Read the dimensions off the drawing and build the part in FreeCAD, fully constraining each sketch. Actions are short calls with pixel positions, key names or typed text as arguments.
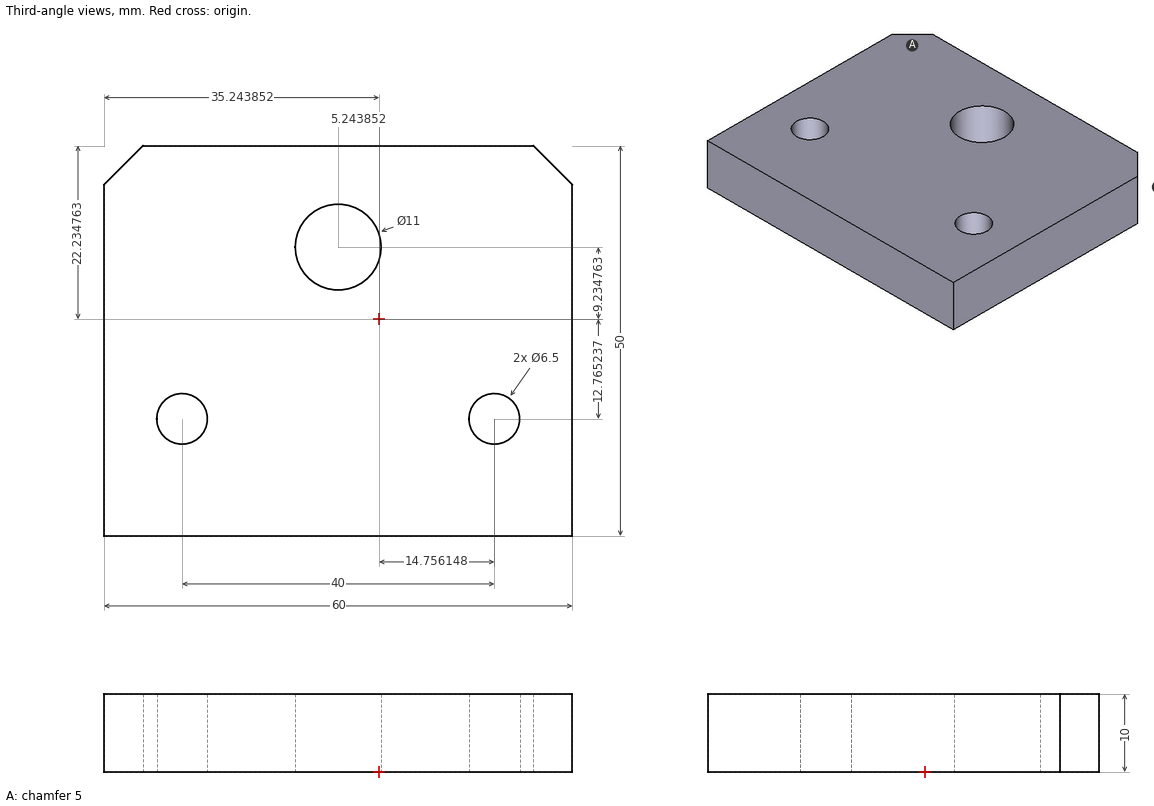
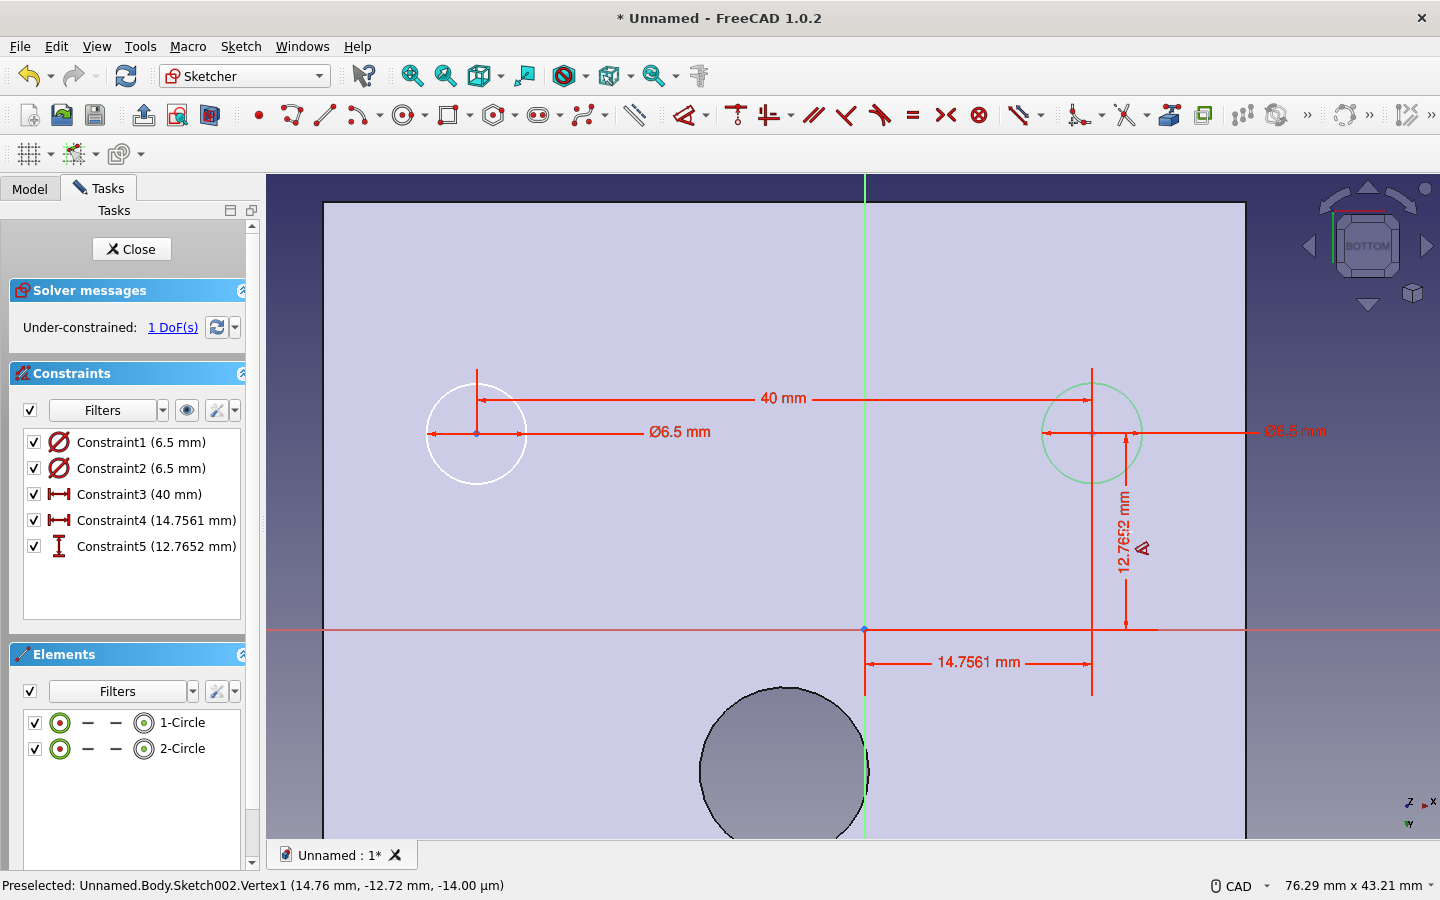
click(477, 434)
click(443, 532)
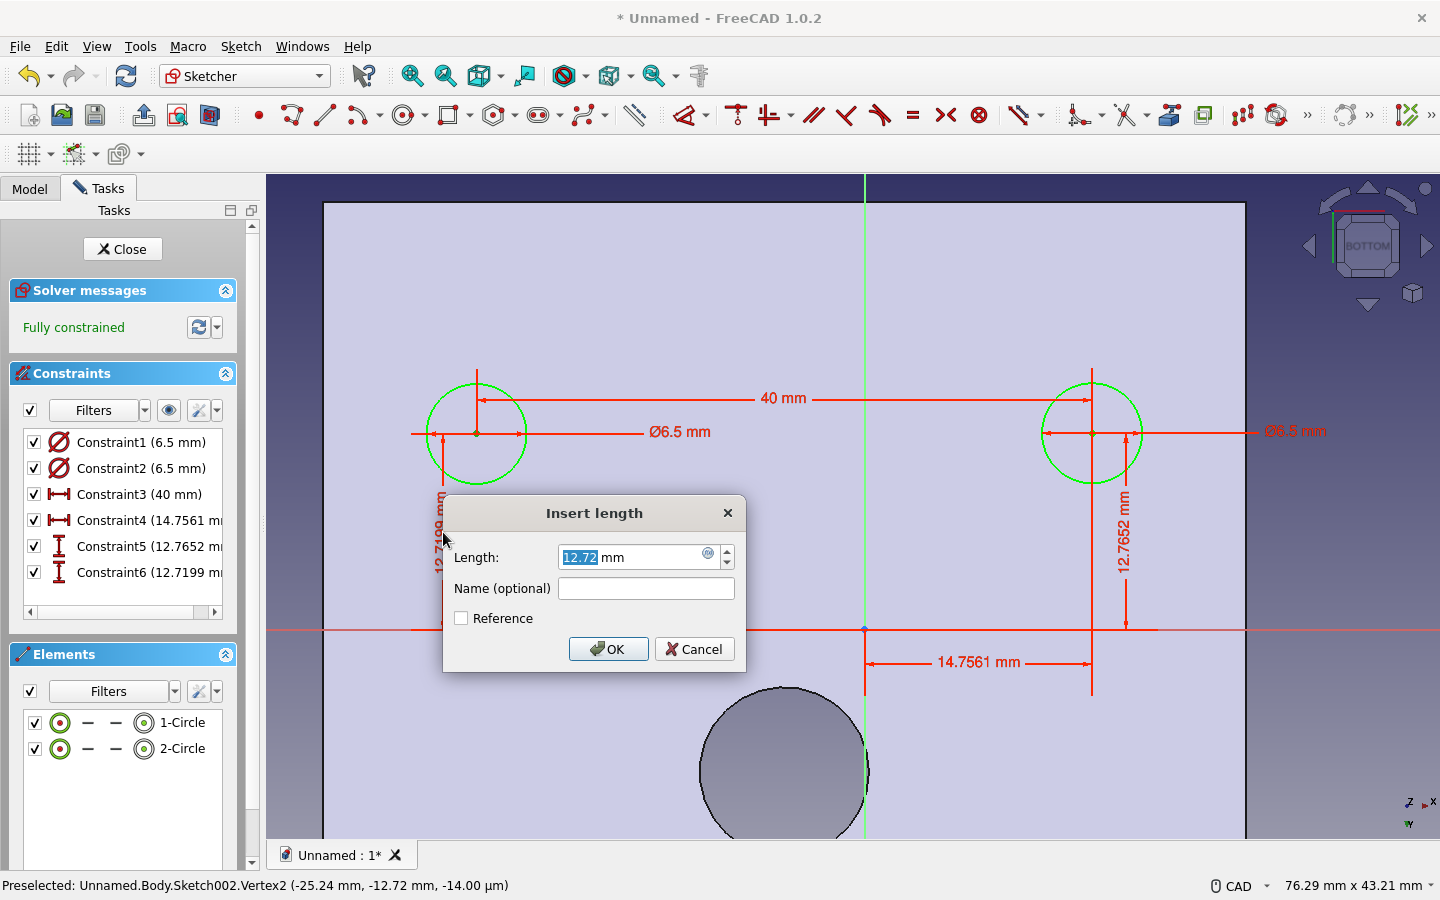
text(12.765237)
key(Return)
key(Escape)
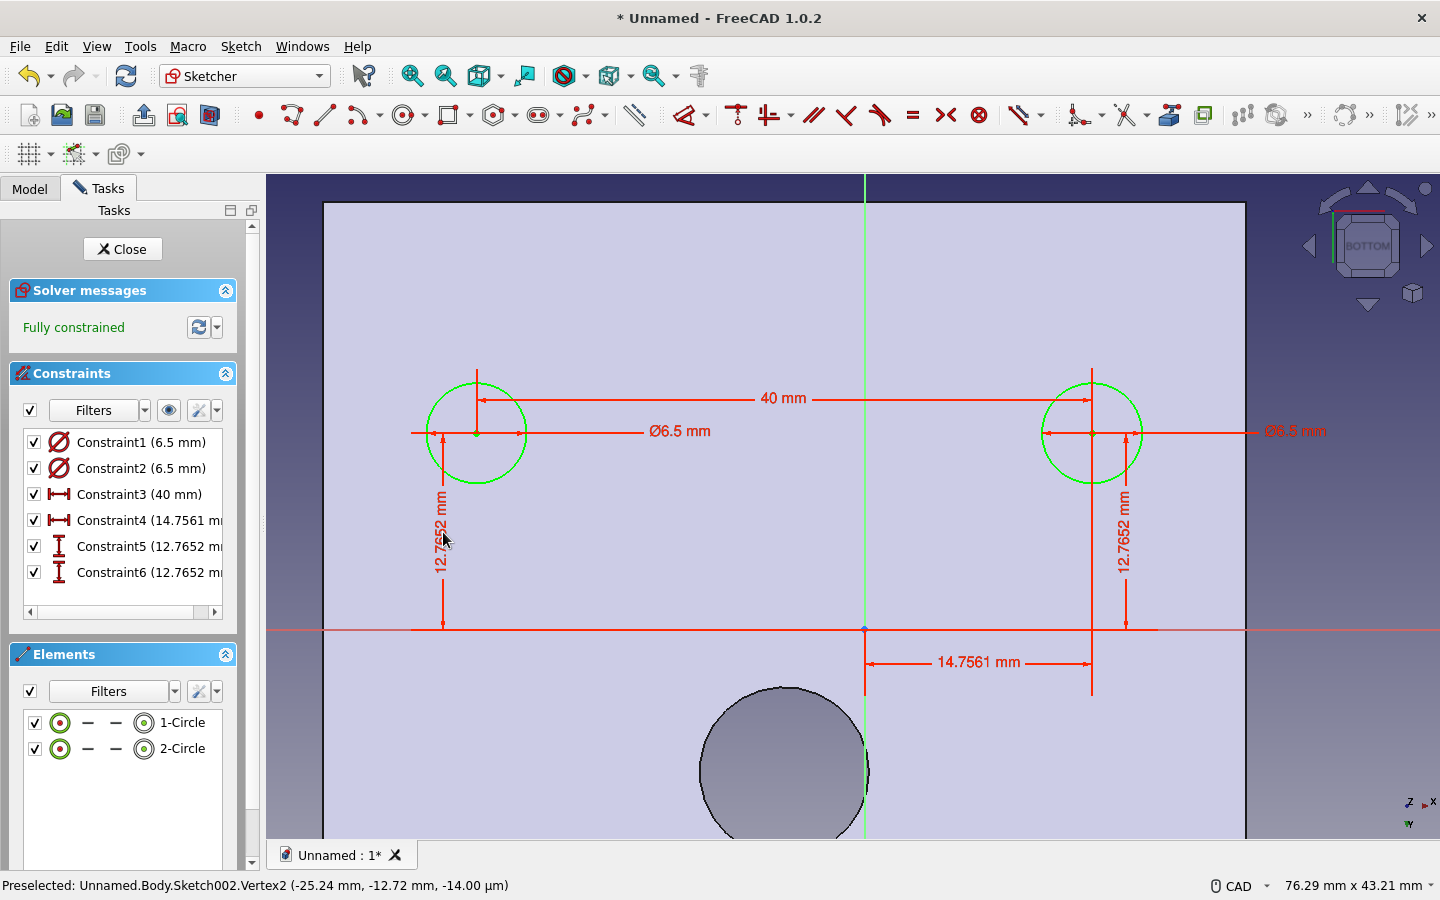
click(123, 249)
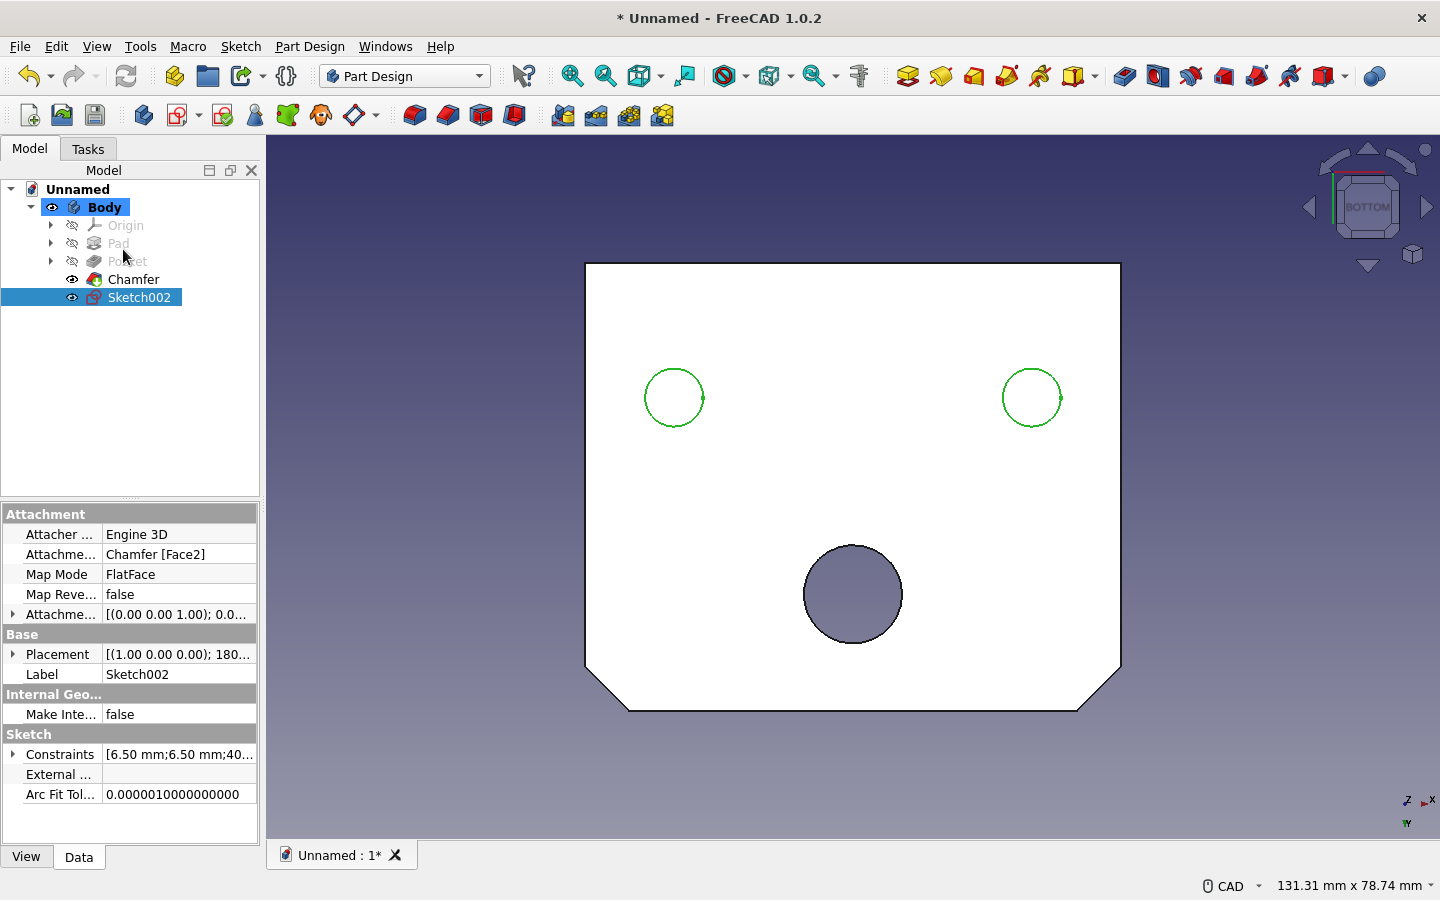
click(1125, 76)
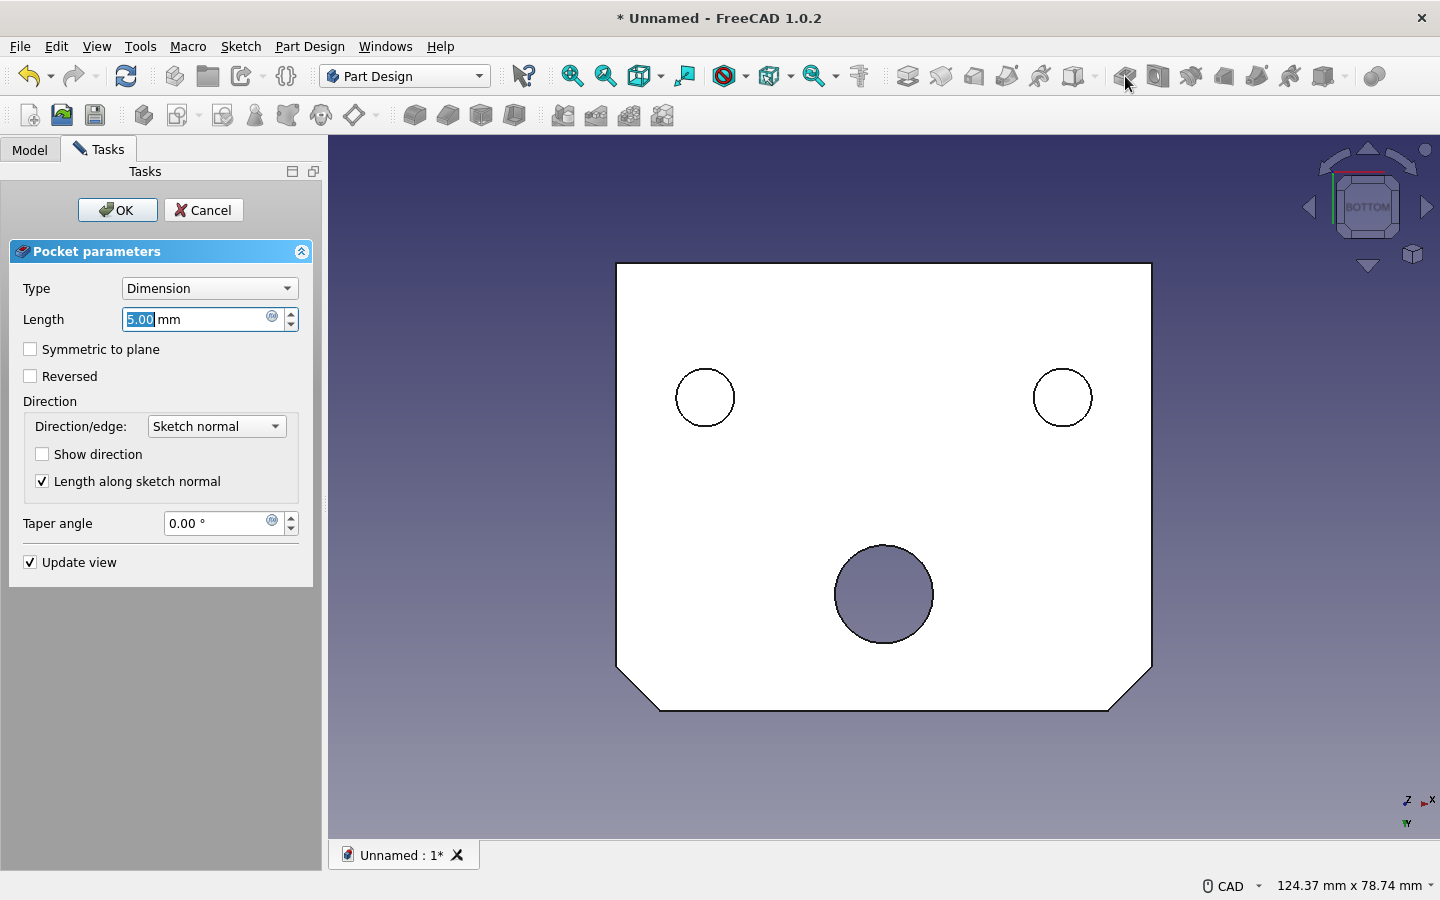
click(210, 288)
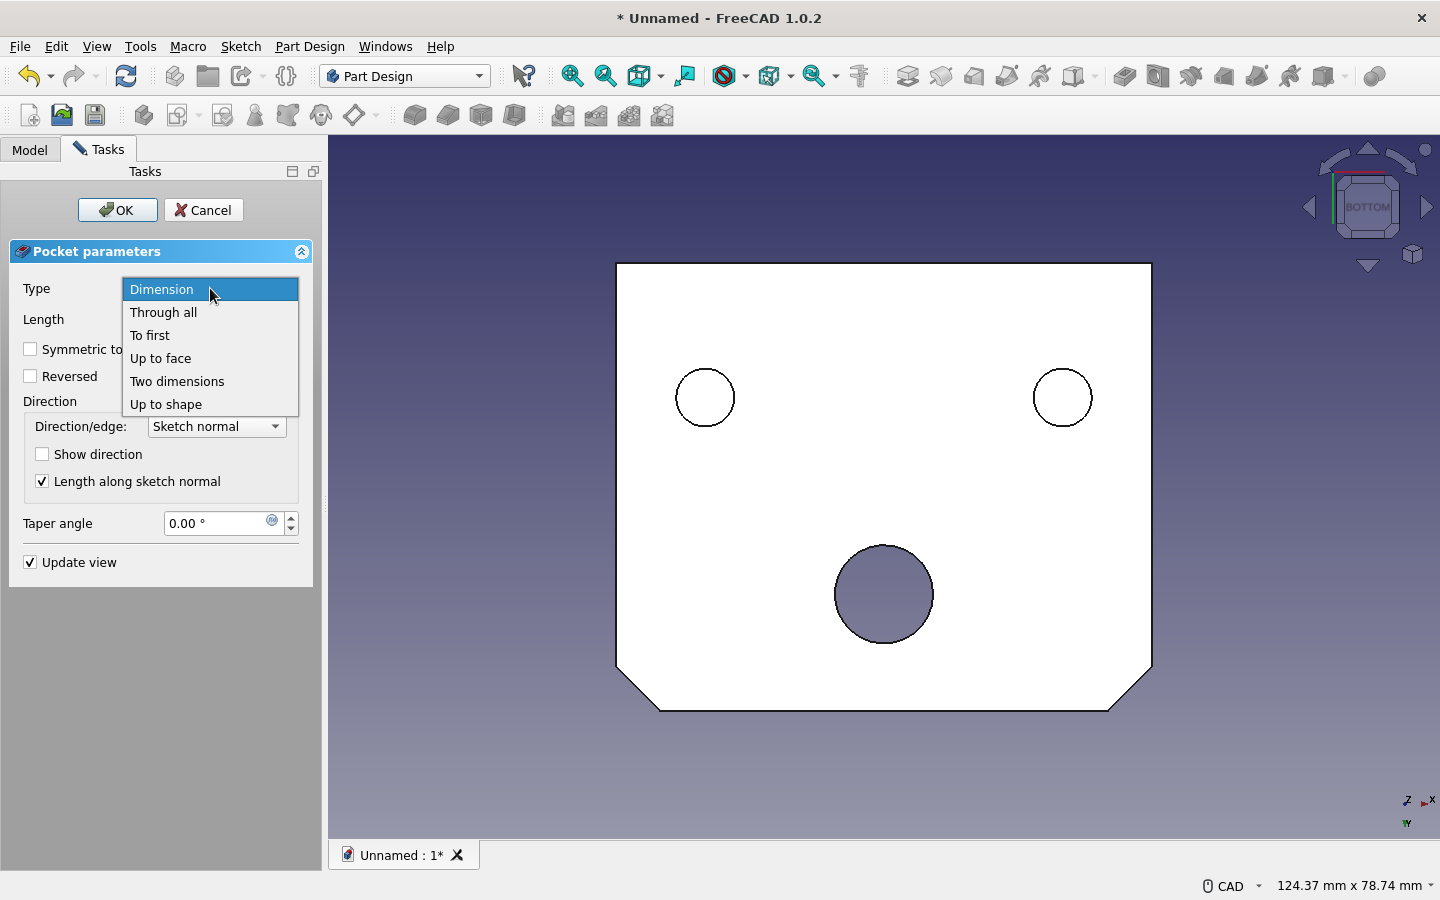
click(208, 312)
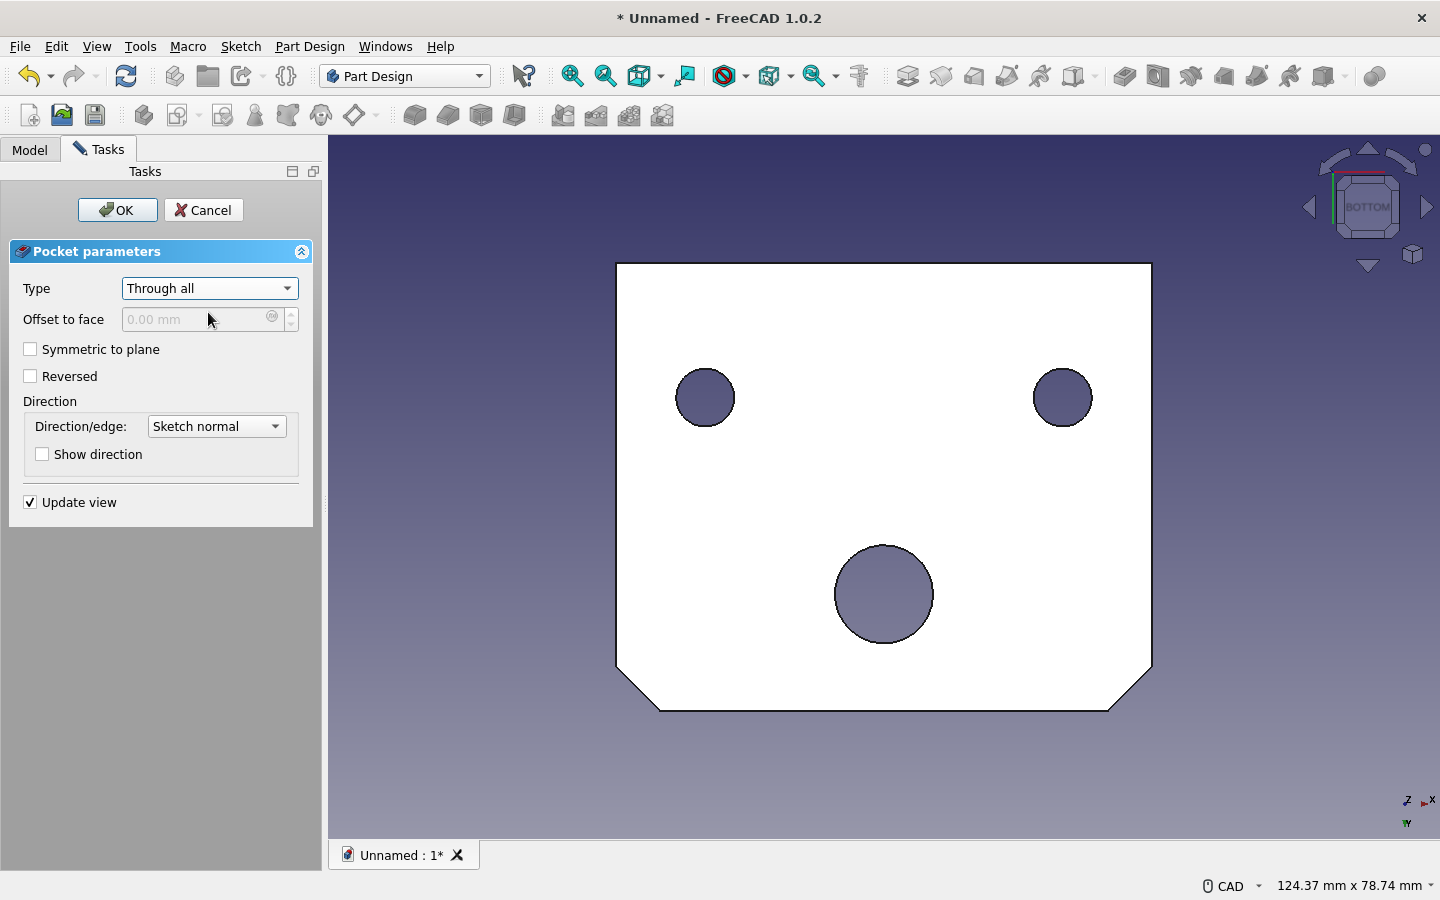
click(118, 210)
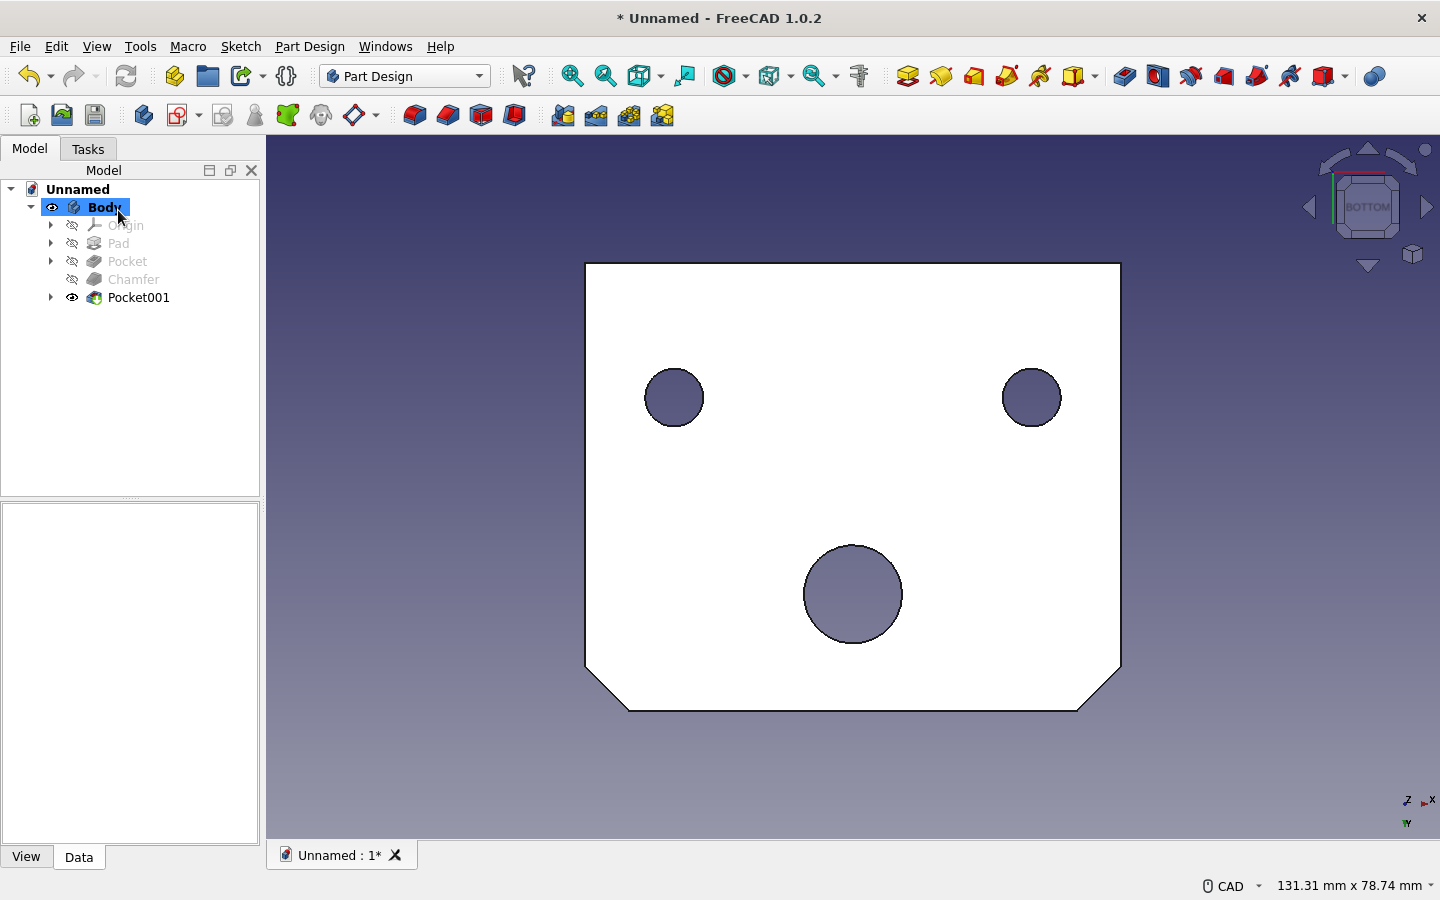
key(0)